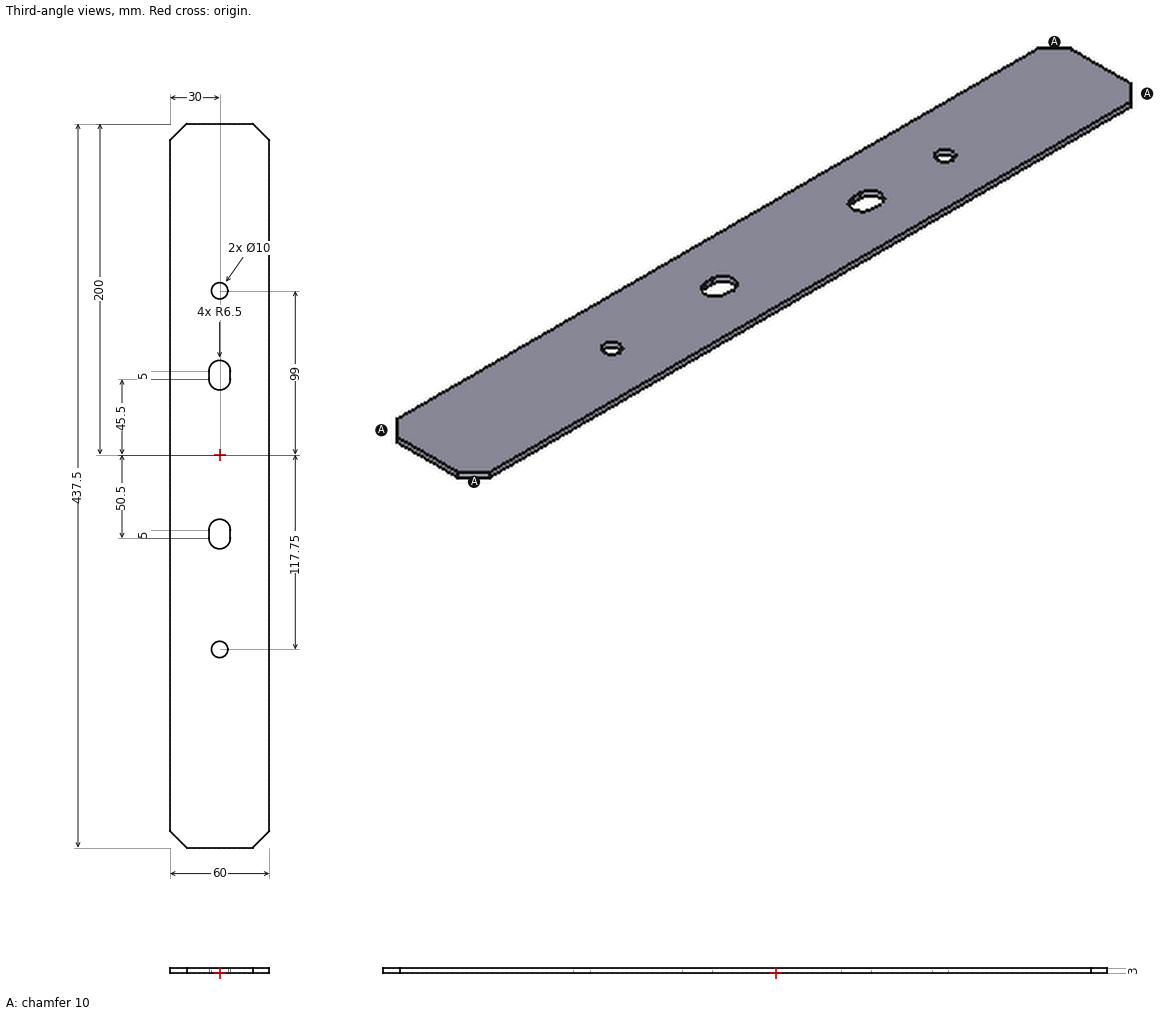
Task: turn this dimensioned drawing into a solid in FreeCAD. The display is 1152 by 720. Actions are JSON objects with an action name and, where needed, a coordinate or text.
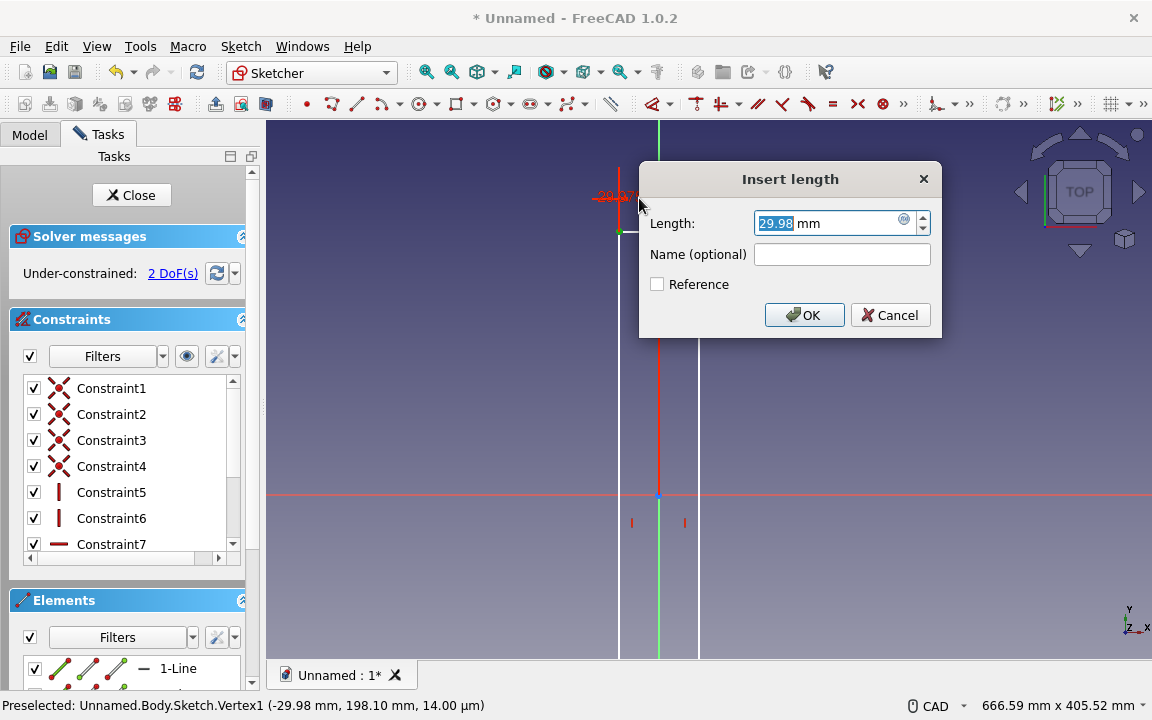
{"action": "type", "text": "30"}
{"action": "key", "text": "Return"}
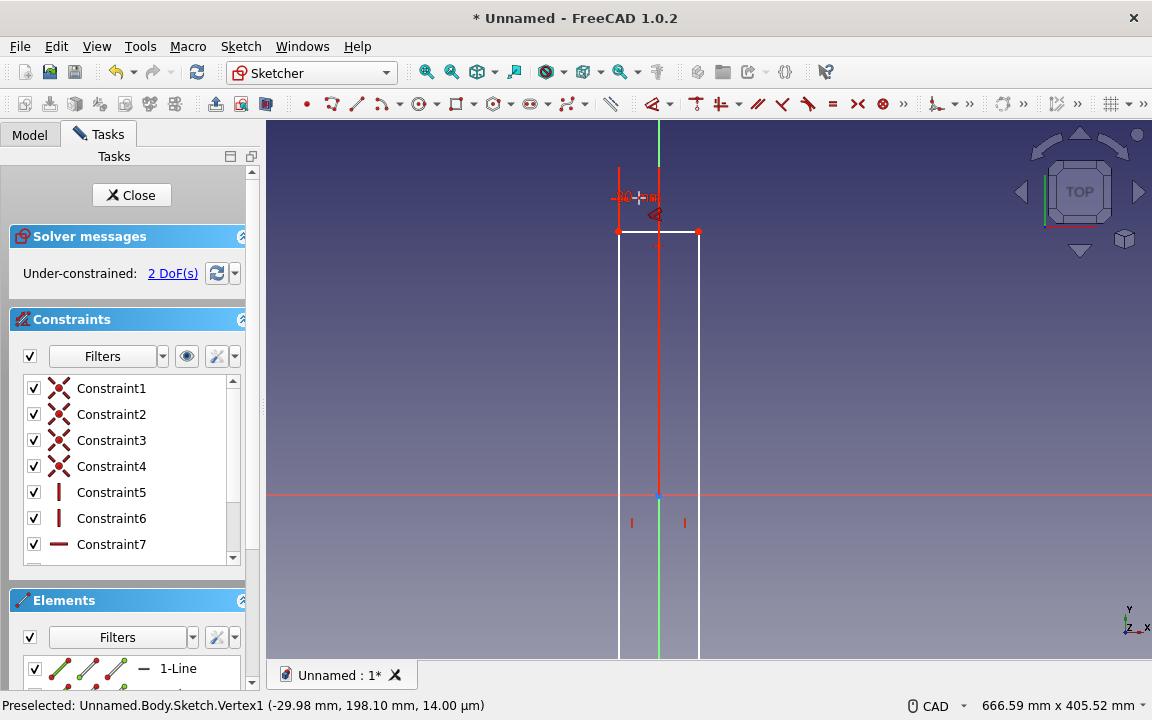
{"action": "left_click", "coordinate": [619, 232]}
{"action": "left_click", "coordinate": [585, 363]}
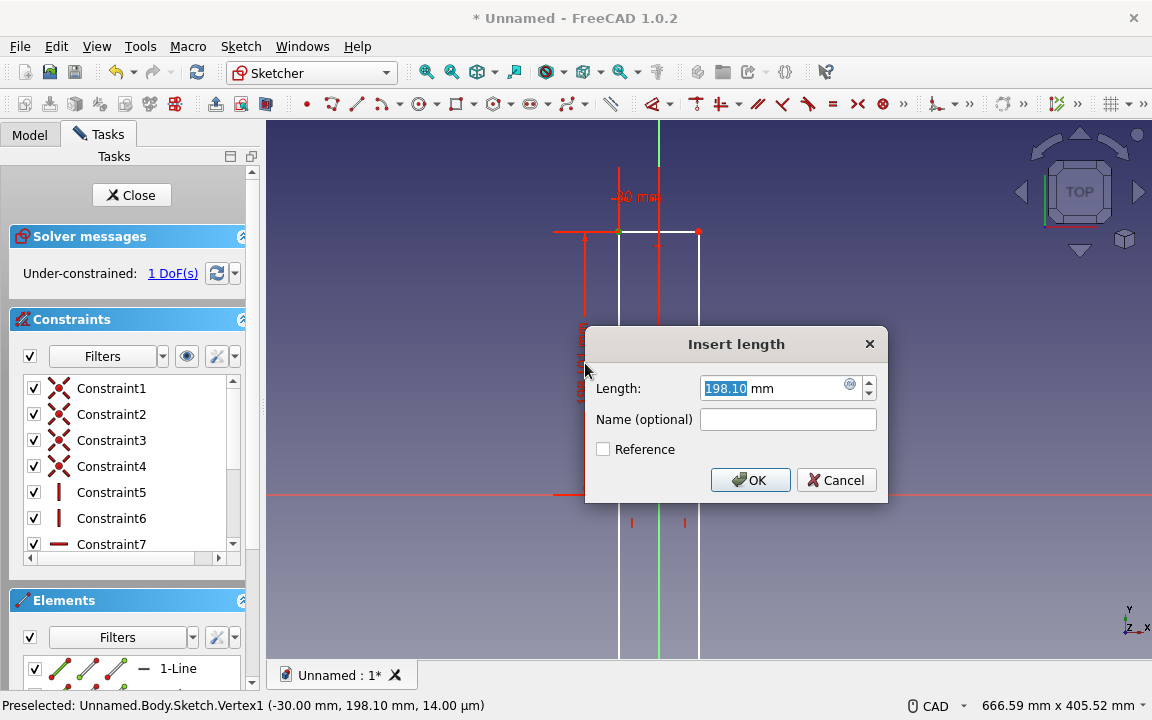
{"action": "type", "text": "200"}
{"action": "key", "text": "Return"}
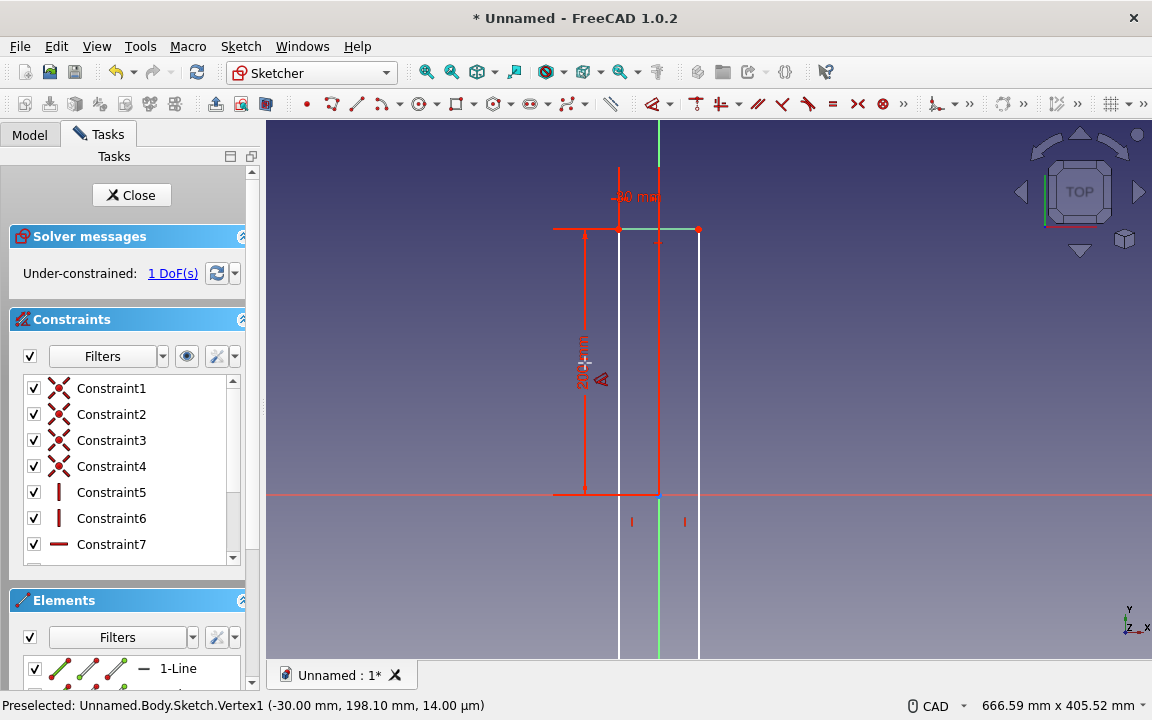
{"action": "left_click", "coordinate": [619, 404]}
{"action": "left_click", "coordinate": [585, 430]}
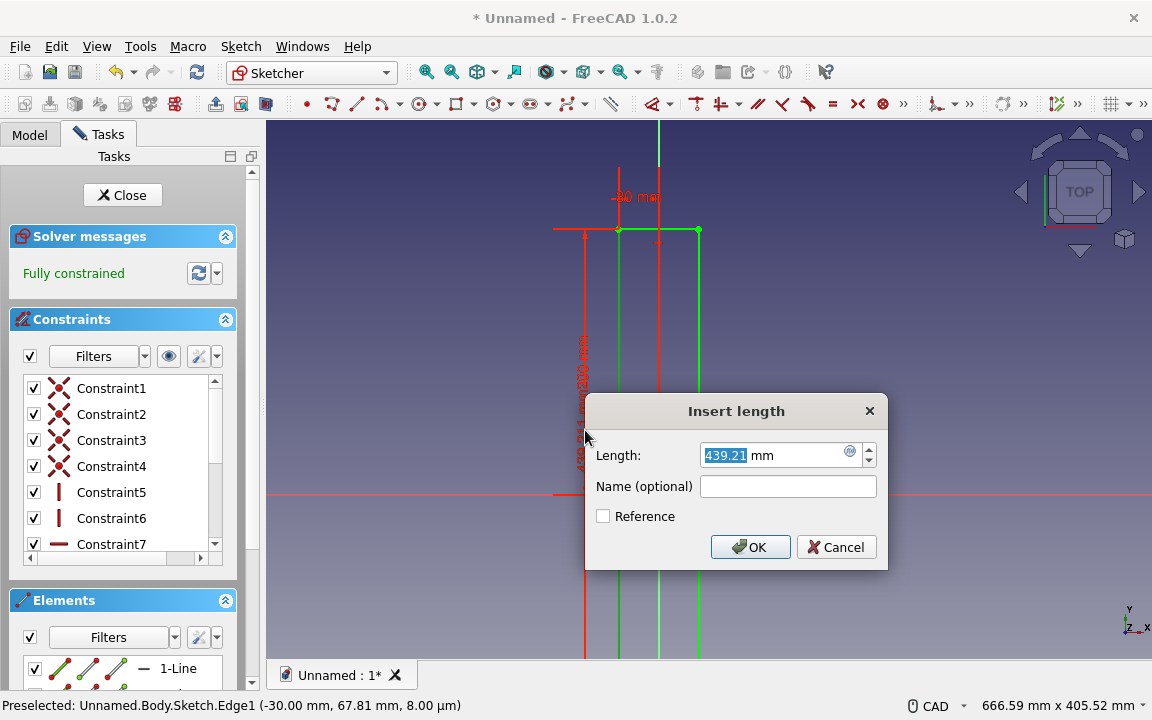
{"action": "type", "text": "437.5"}
{"action": "key", "text": "Return"}
{"action": "key", "text": "Escape"}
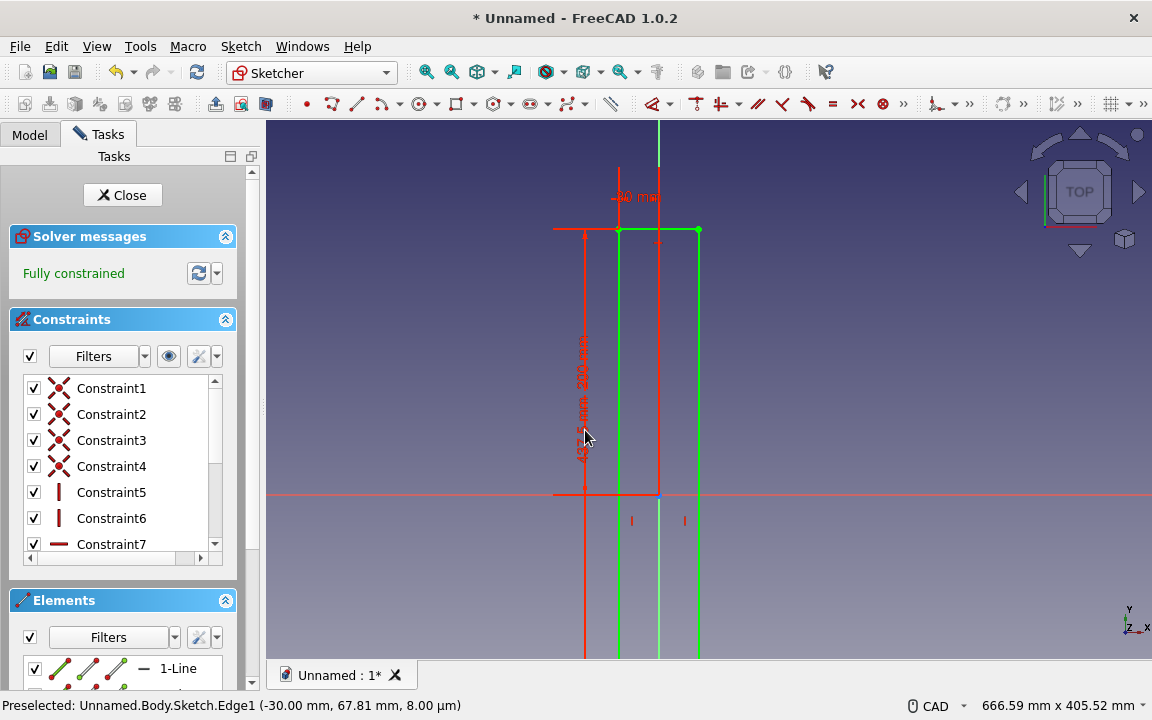
{"action": "left_click", "coordinate": [123, 195]}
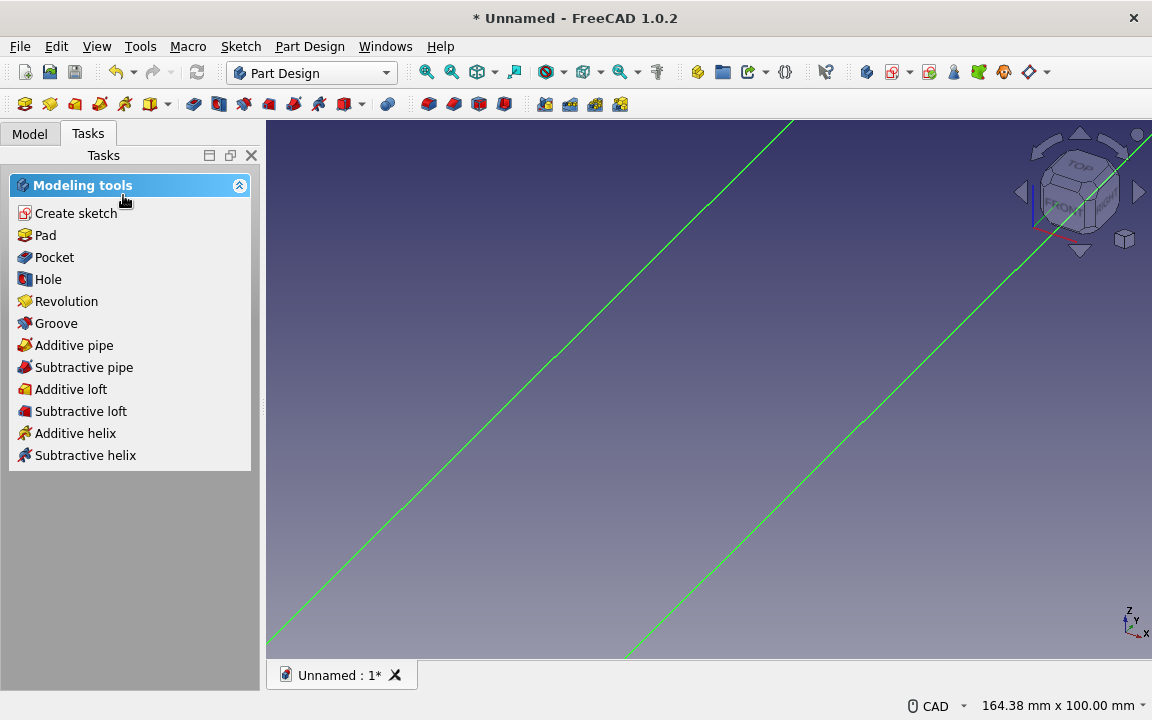
{"action": "left_click", "coordinate": [25, 104]}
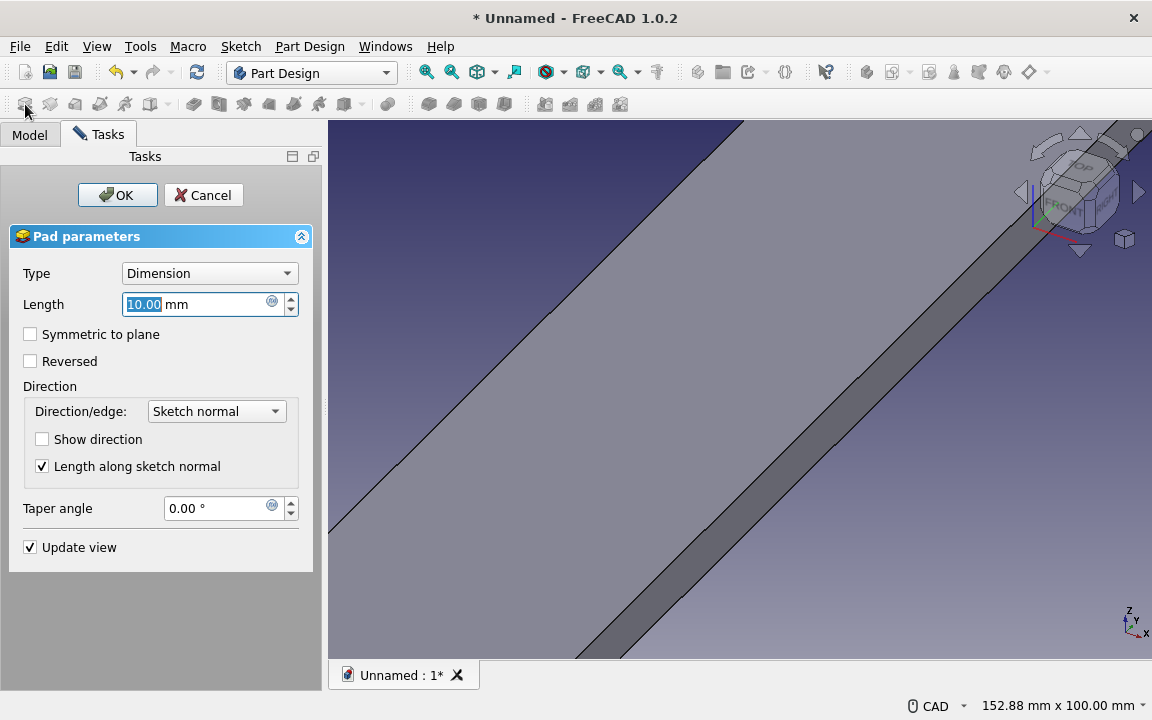
{"action": "type", "text": "3"}
{"action": "key", "text": "Tab"}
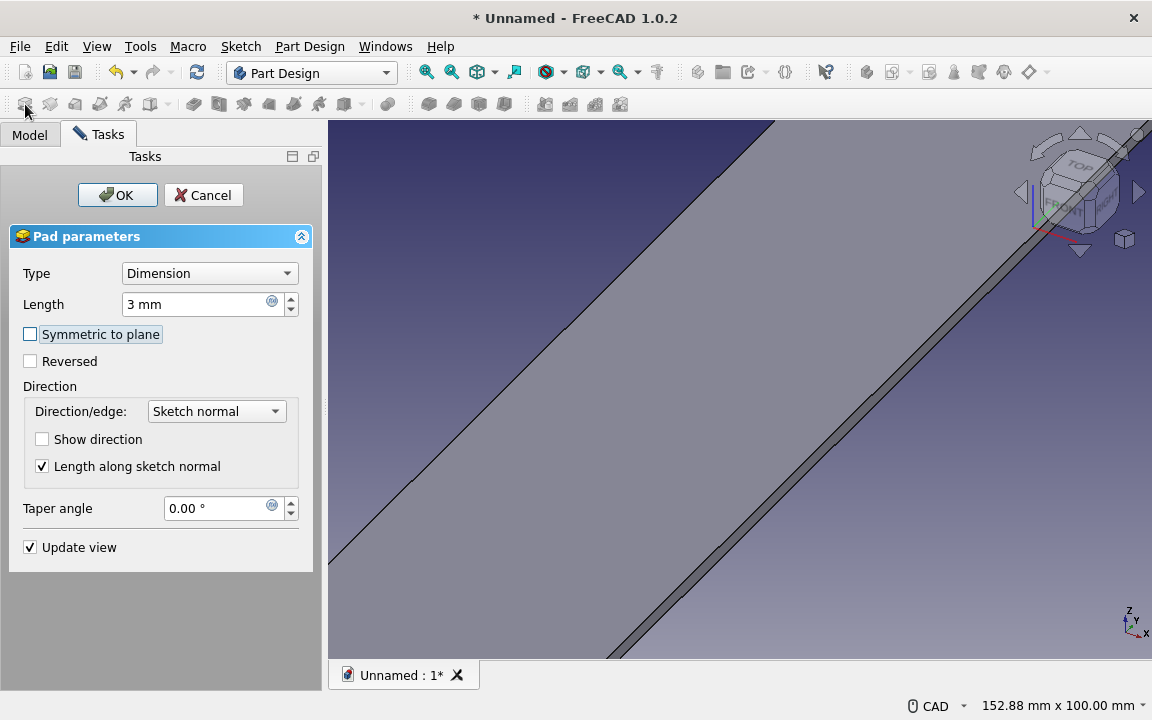
{"action": "left_click", "coordinate": [118, 195]}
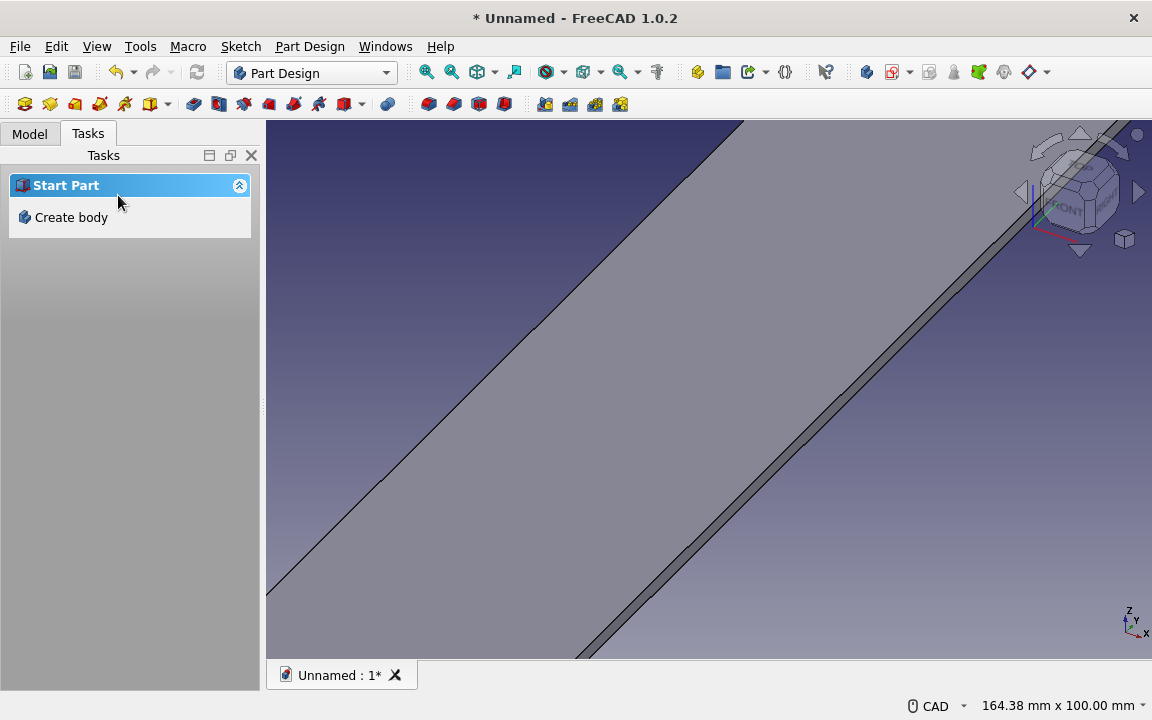
{"action": "left_click", "coordinate": [427, 72]}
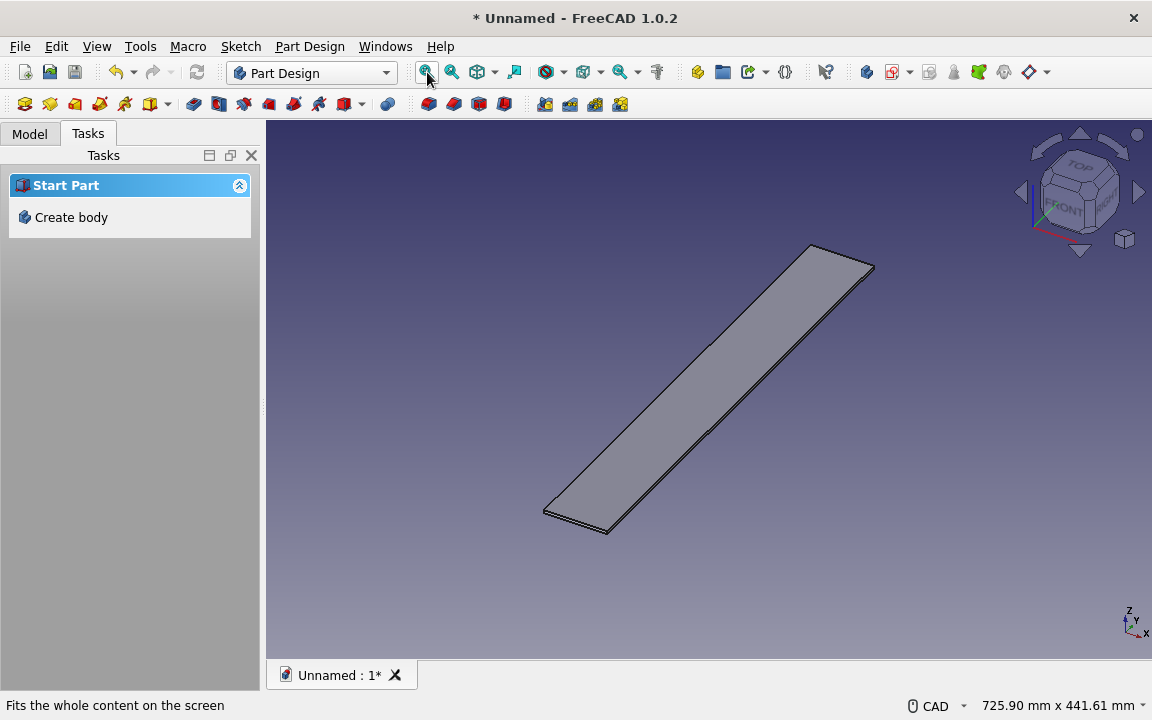
{"action": "scroll", "coordinate": [607, 532], "scroll_direction": "up", "scroll_amount": 12}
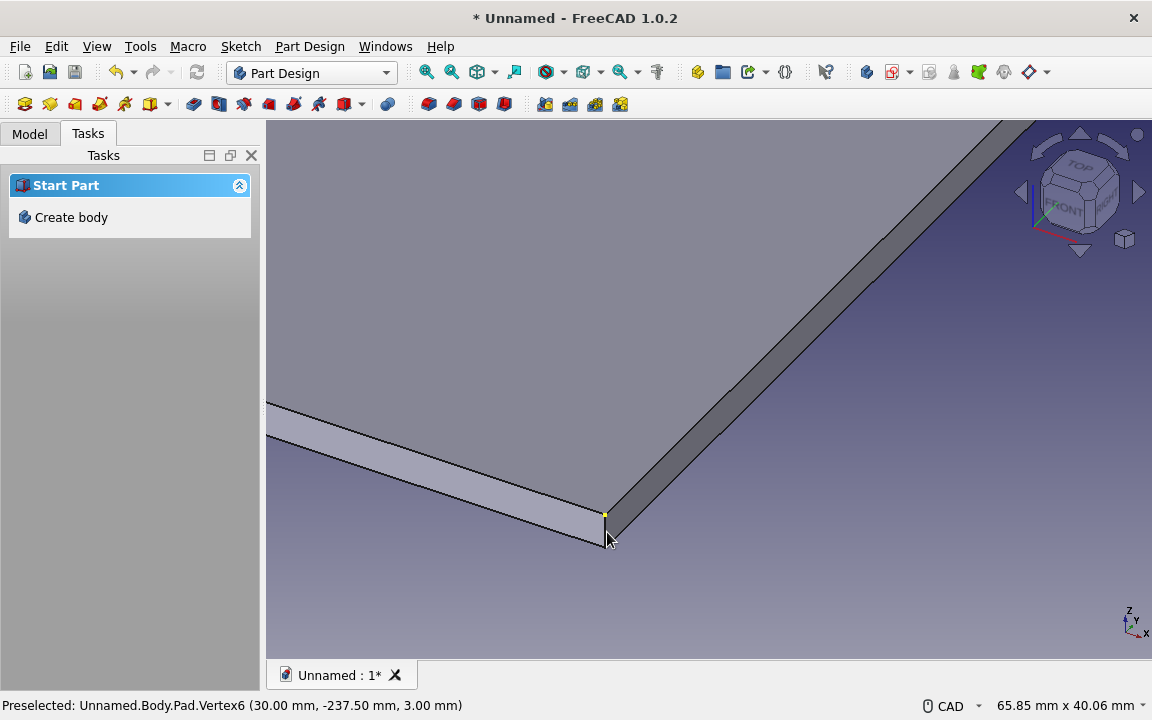
{"action": "left_click", "coordinate": [605, 530]}